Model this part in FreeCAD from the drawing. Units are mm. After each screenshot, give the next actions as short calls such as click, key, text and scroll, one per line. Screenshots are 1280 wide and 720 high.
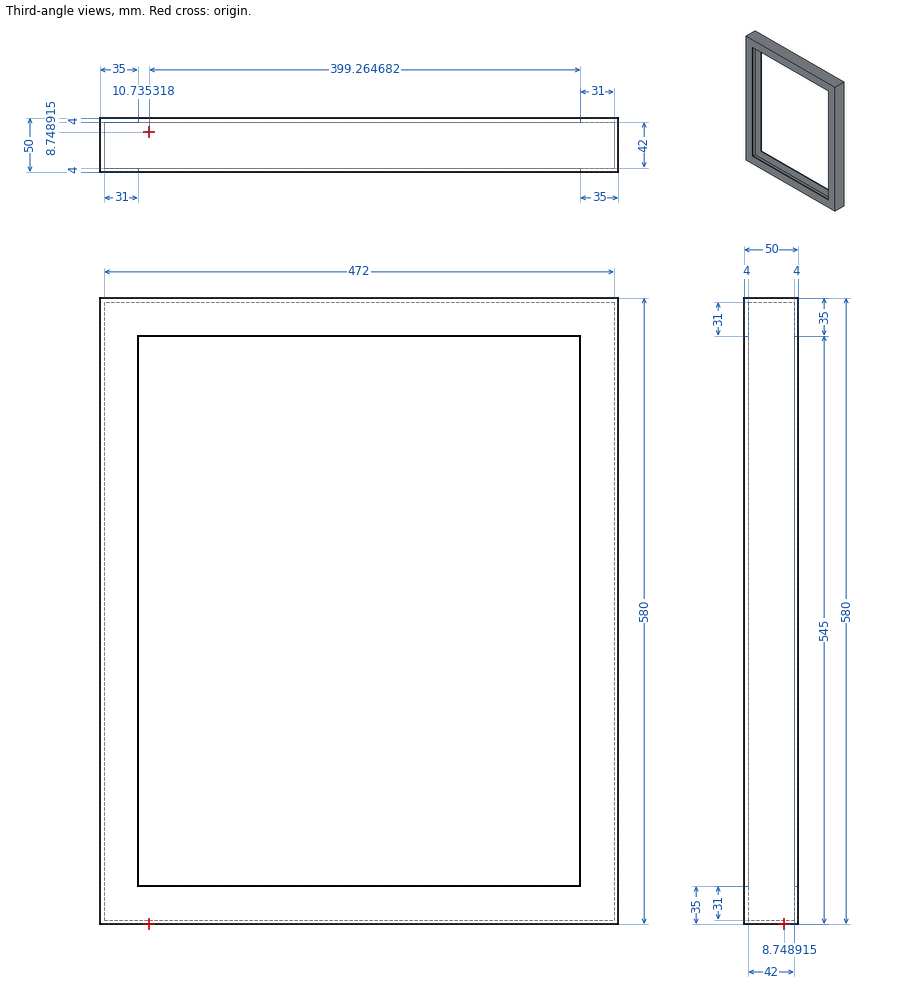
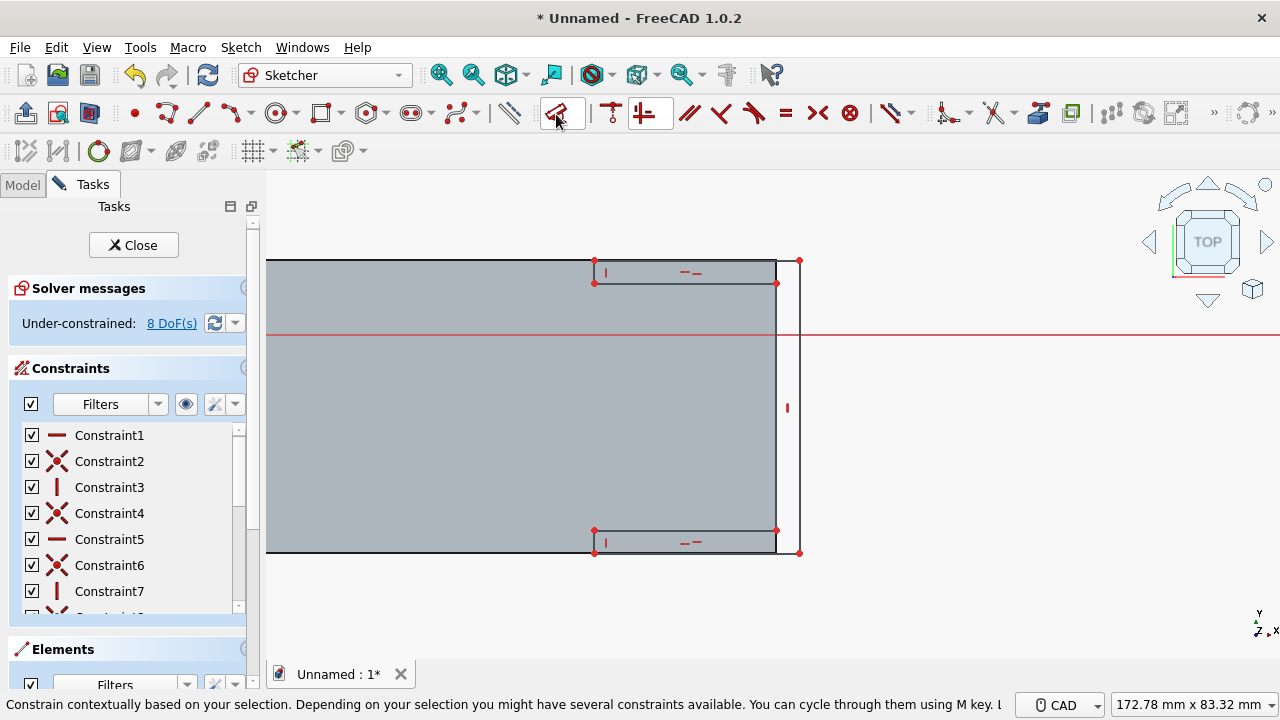
scroll(594, 540, up, 3)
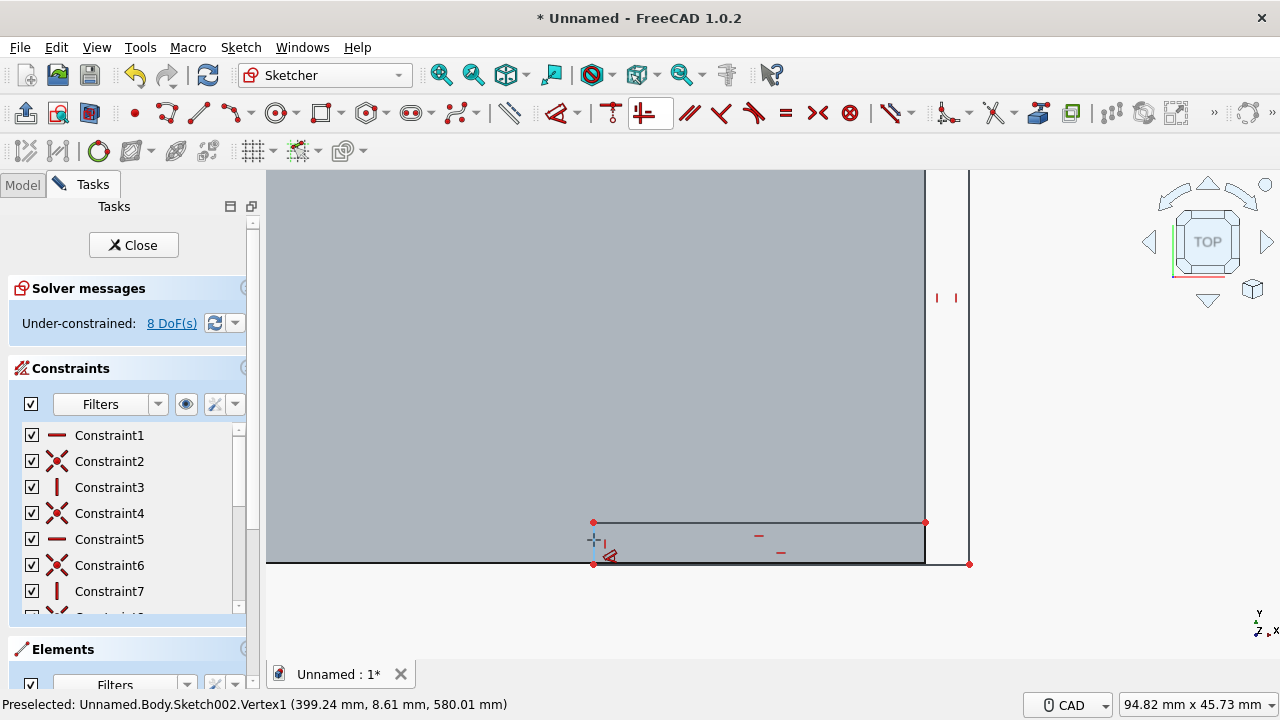
click(594, 540)
click(560, 544)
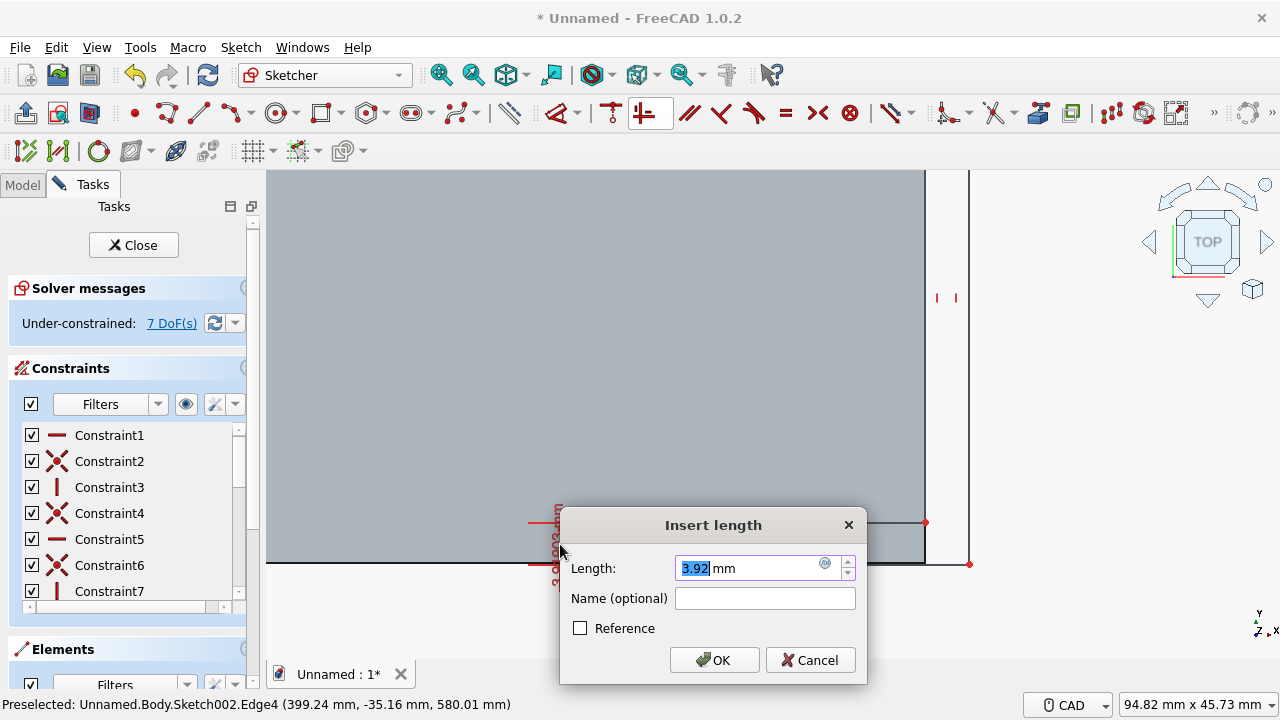
text(4)
key(Return)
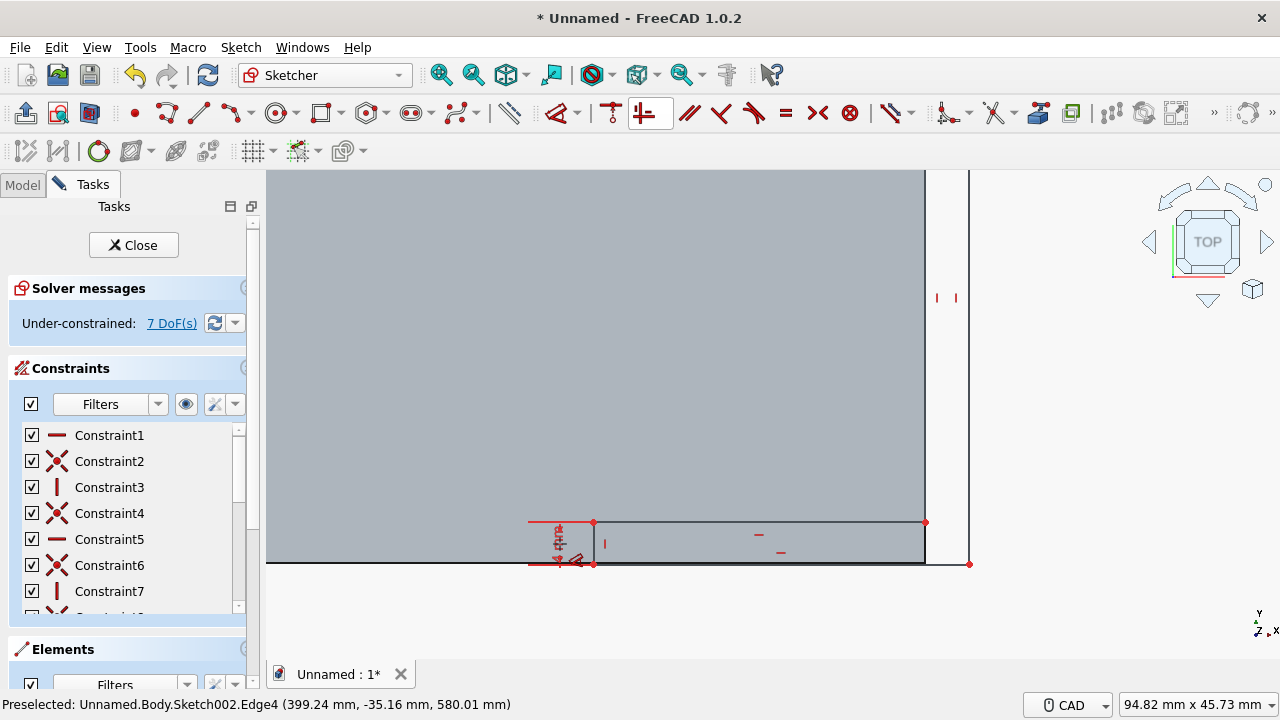
scroll(611, 559, down, 3)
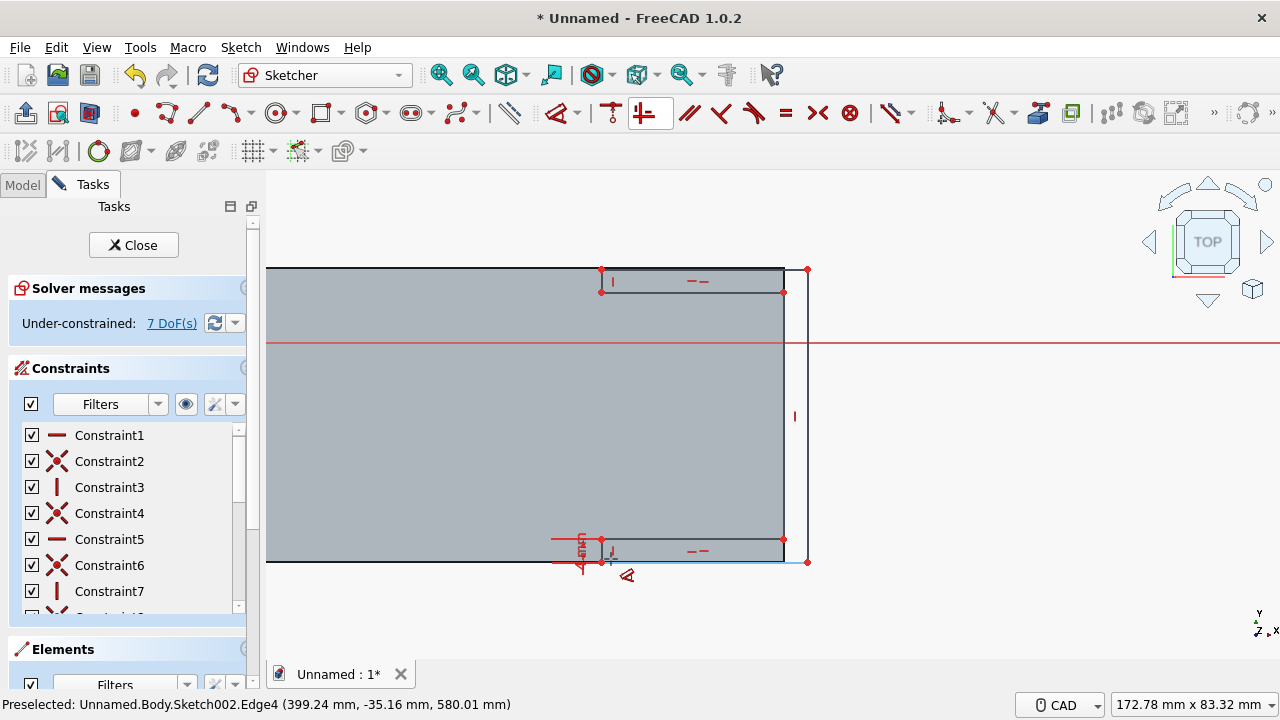
scroll(602, 276, up, 4)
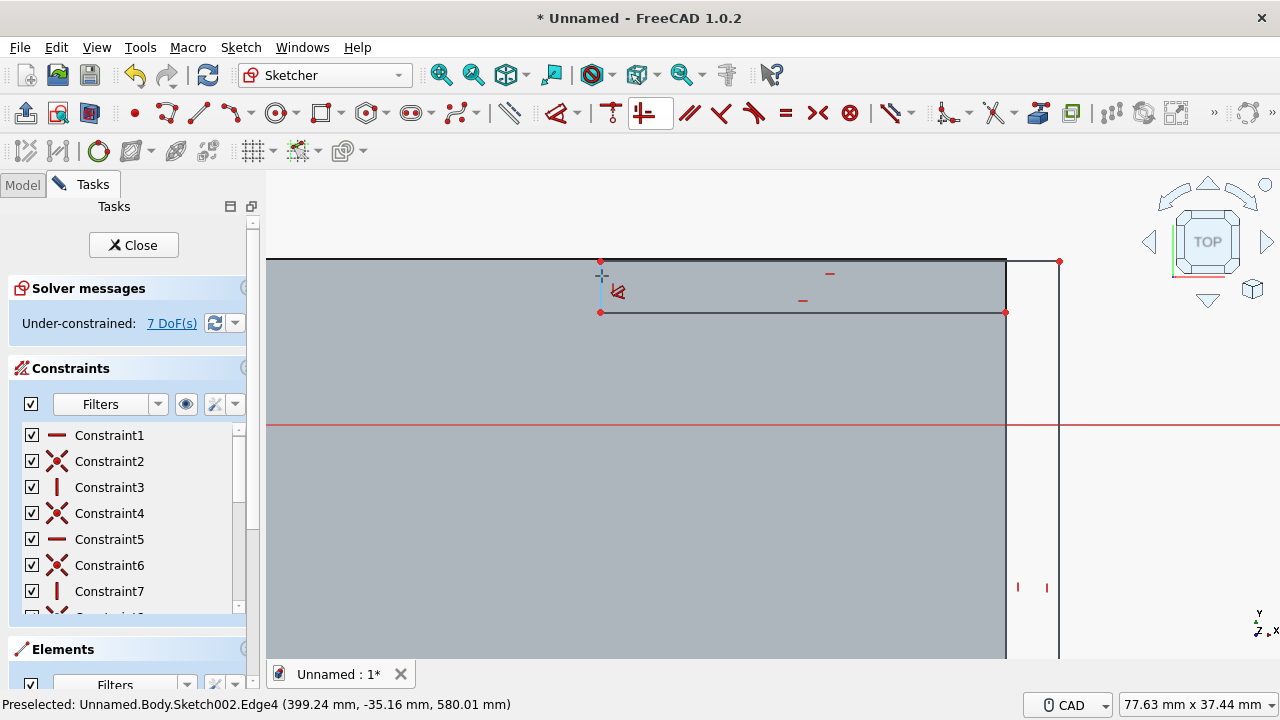
click(601, 277)
click(567, 287)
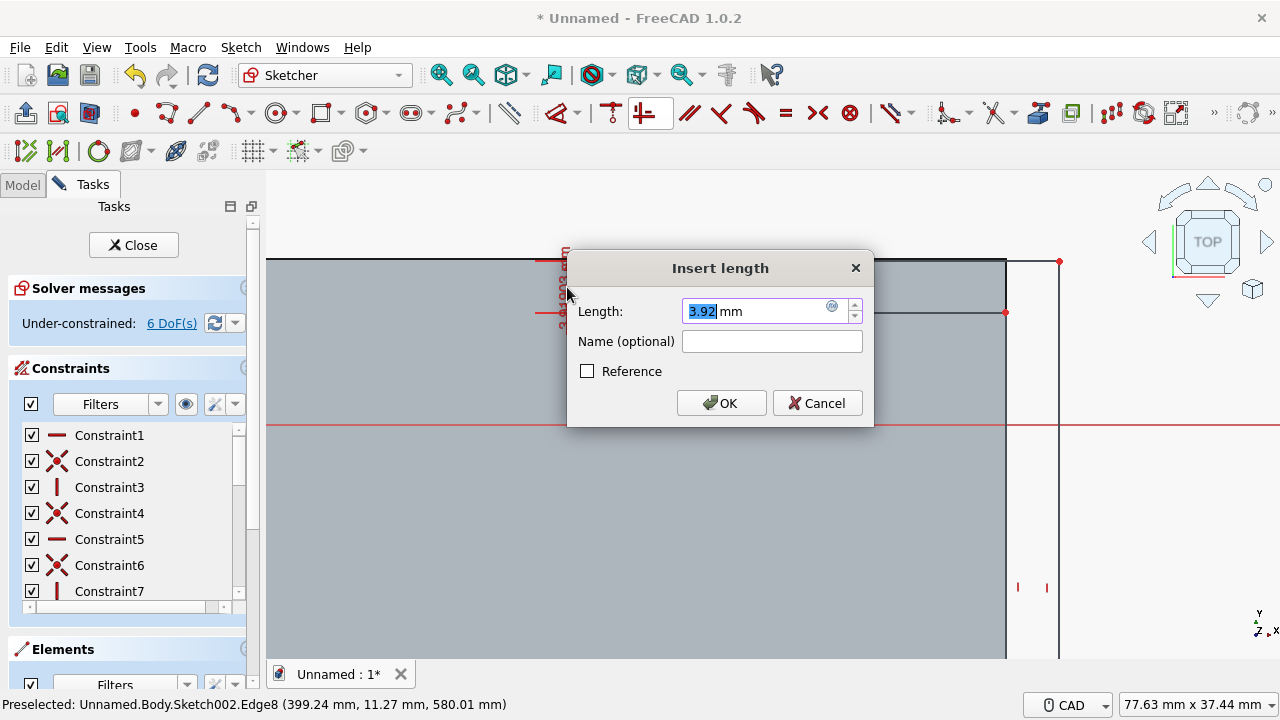
text(4)
key(Return)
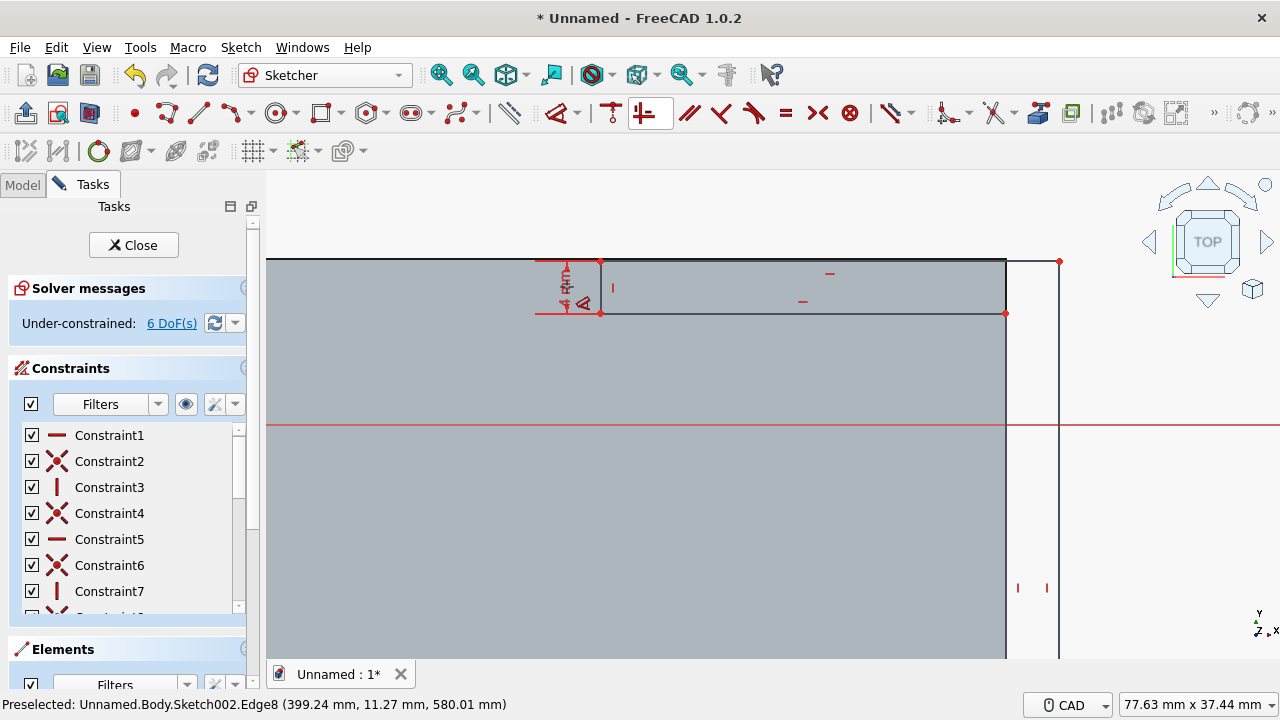
click(722, 314)
click(803, 280)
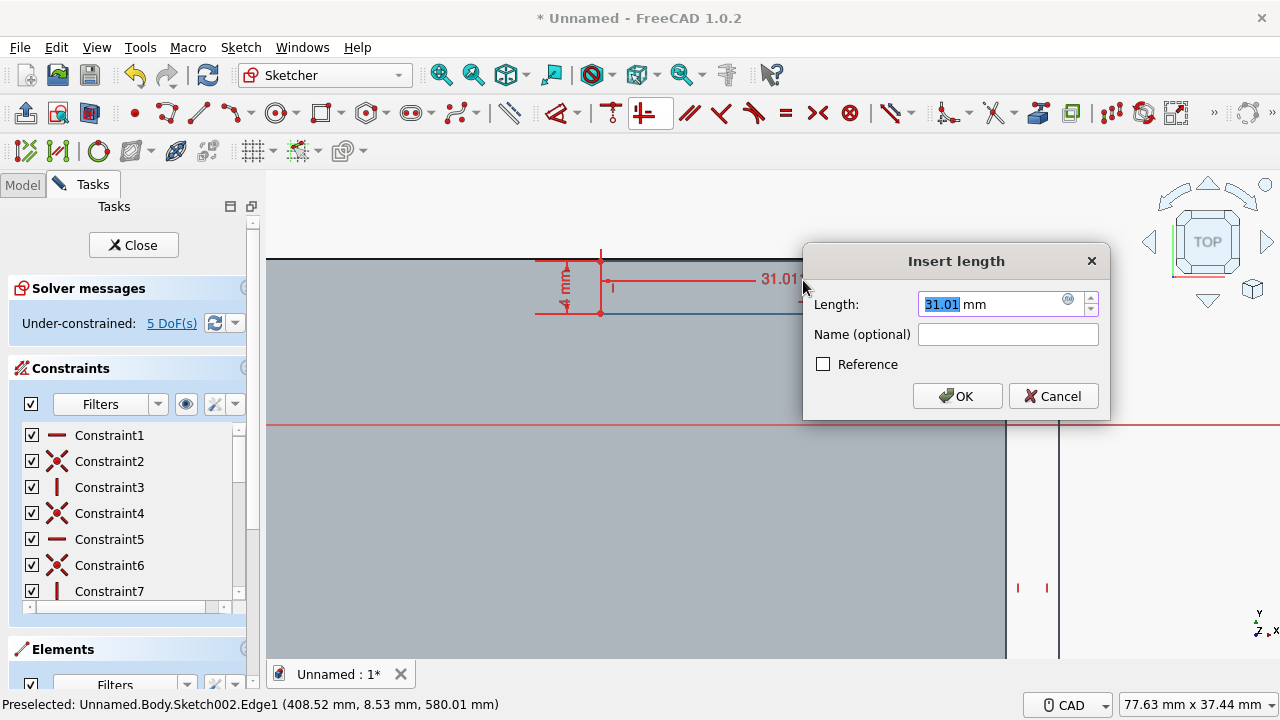
text(31)
key(Return)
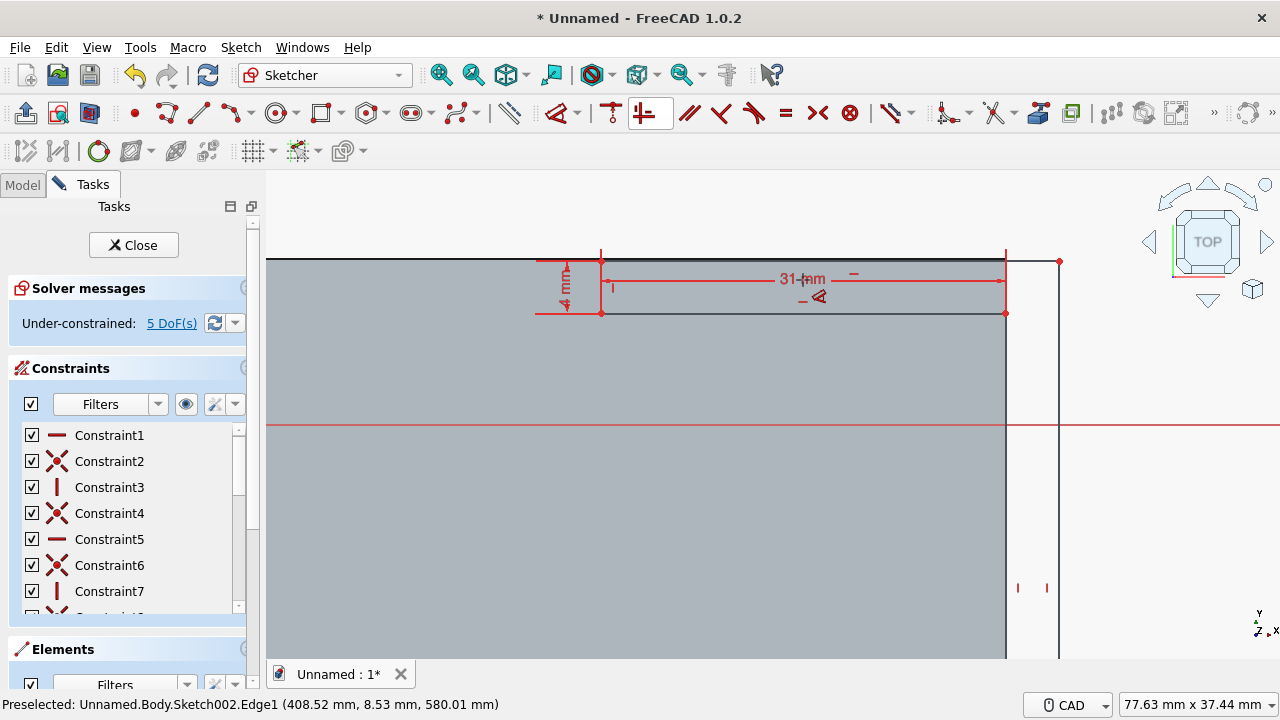
click(1006, 478)
click(1040, 472)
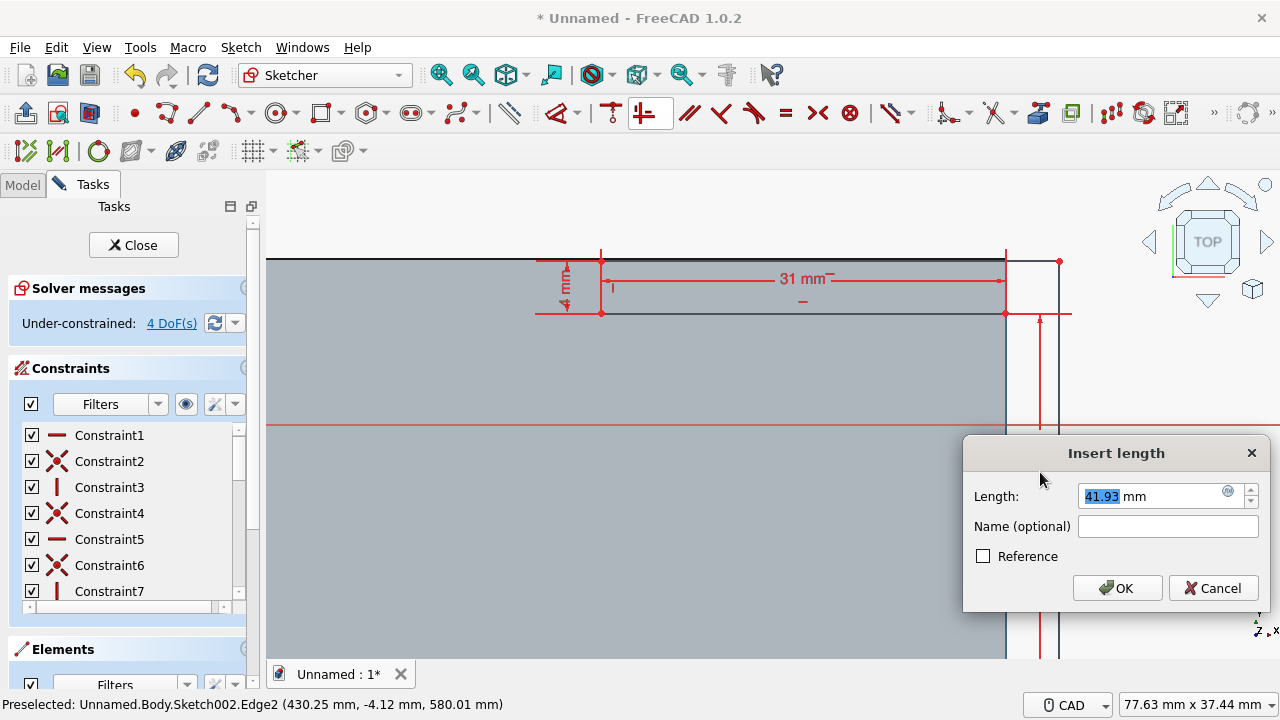
text(42)
key(Return)